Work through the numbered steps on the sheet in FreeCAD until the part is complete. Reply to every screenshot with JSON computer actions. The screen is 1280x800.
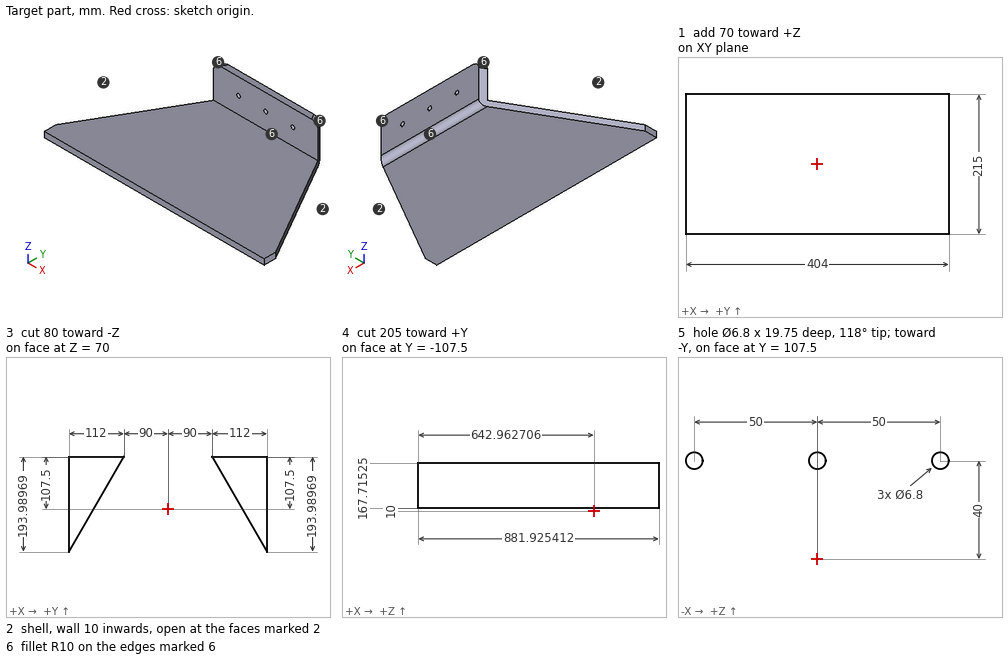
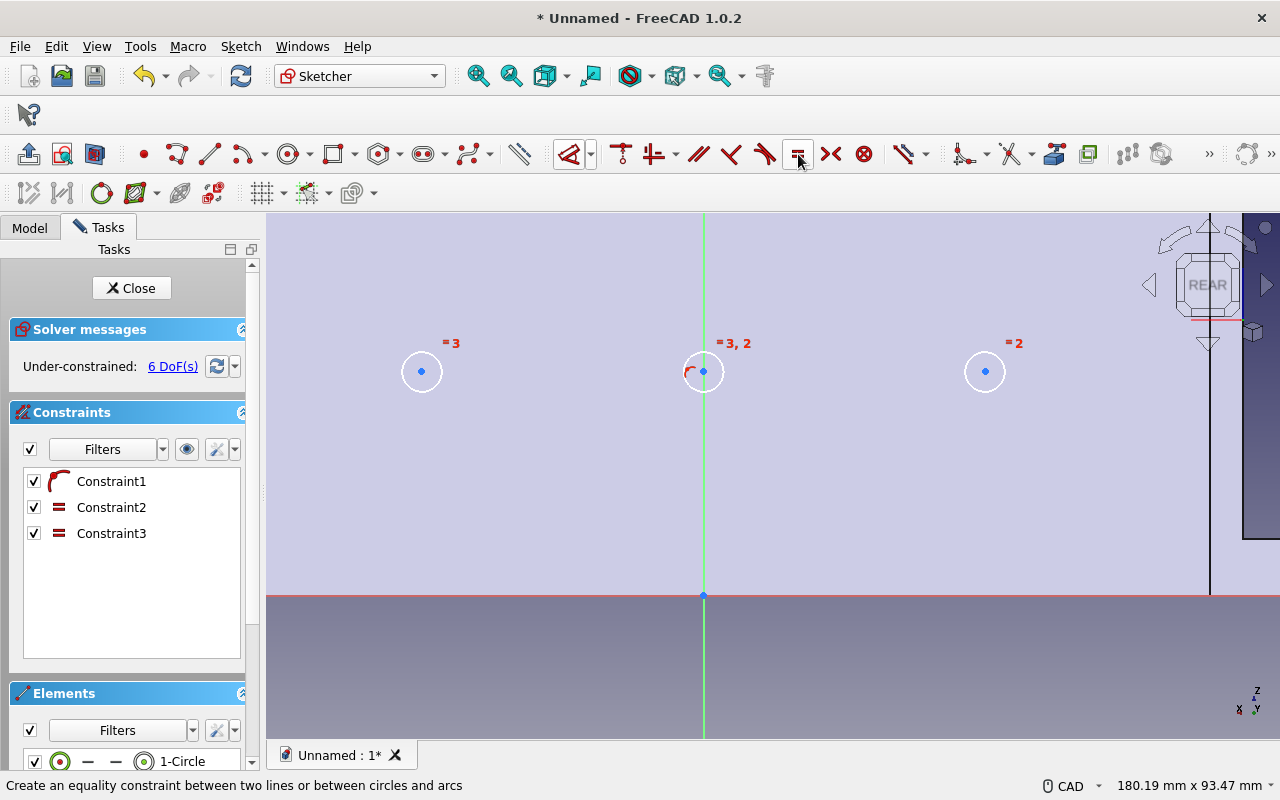
{"action": "left_click", "coordinate": [985, 372]}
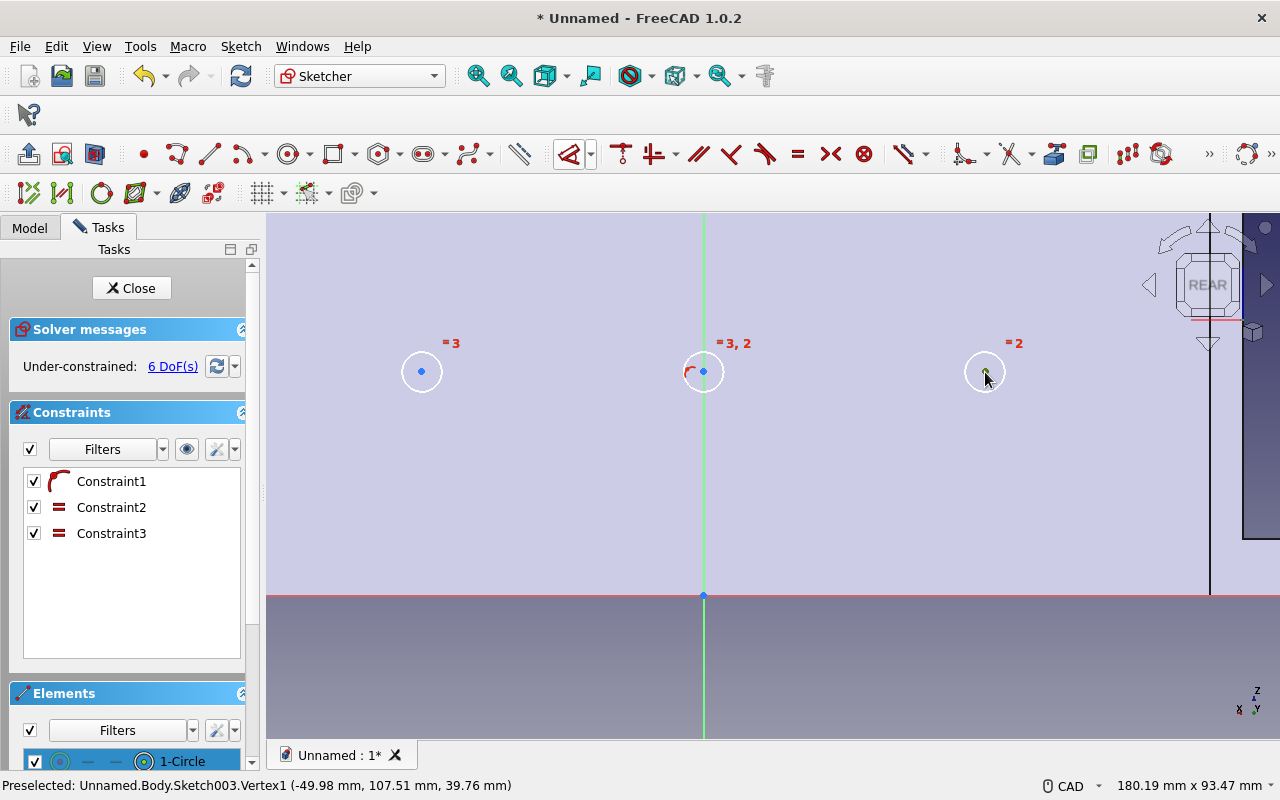
{"action": "left_click", "coordinate": [704, 372]}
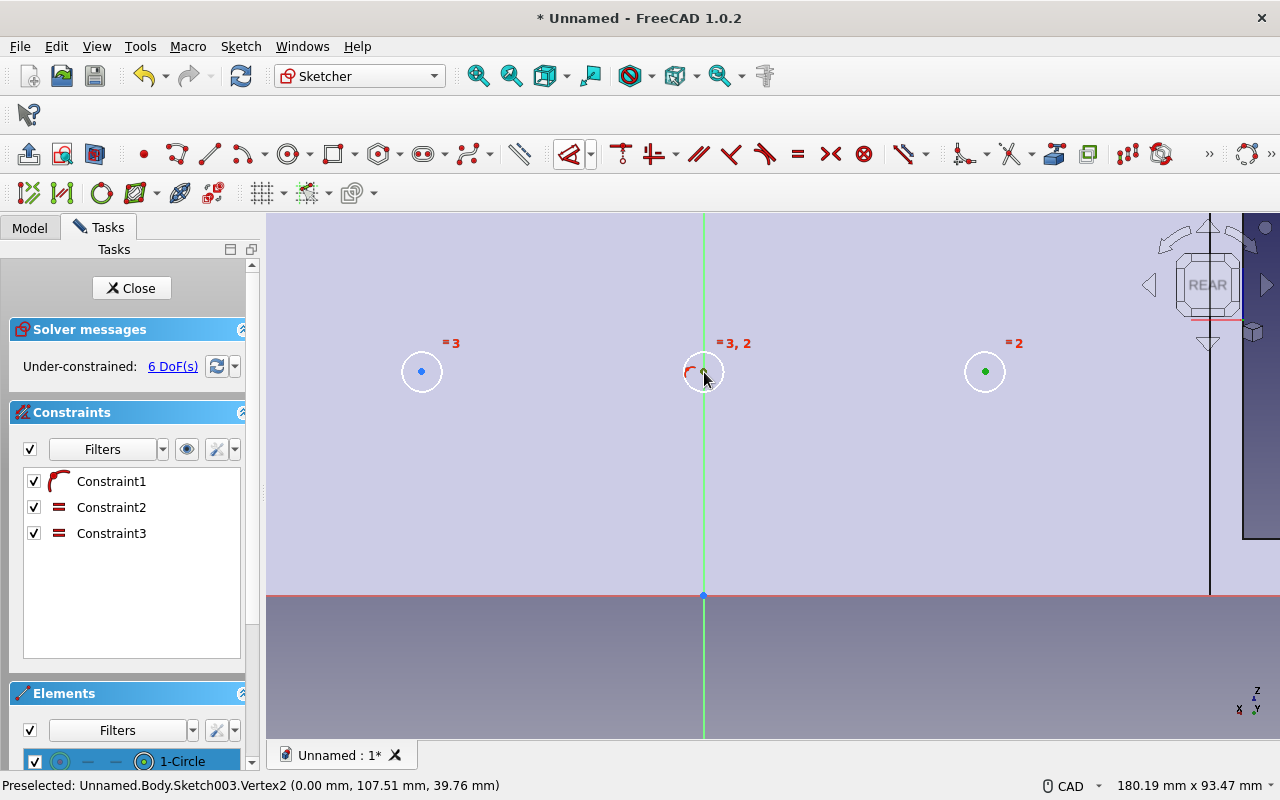
{"action": "left_click", "coordinate": [676, 154]}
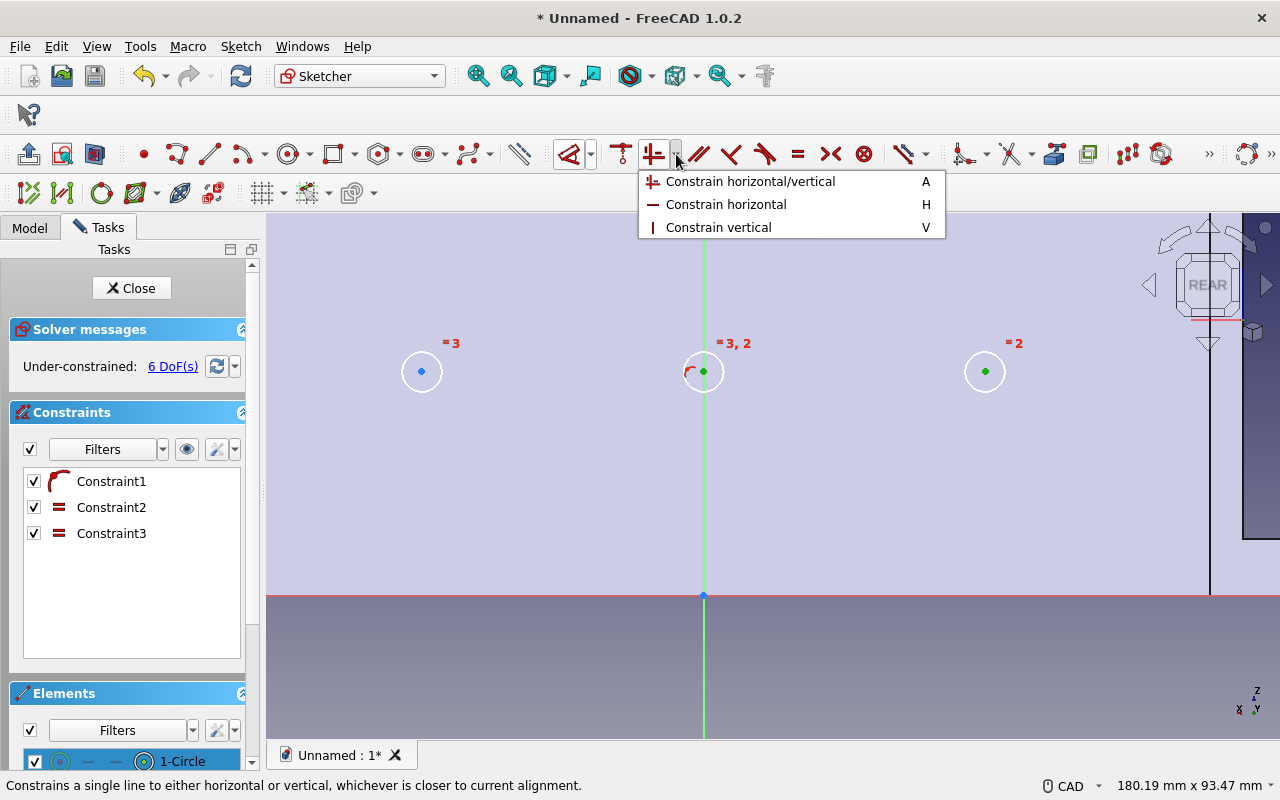
{"action": "left_click", "coordinate": [792, 204]}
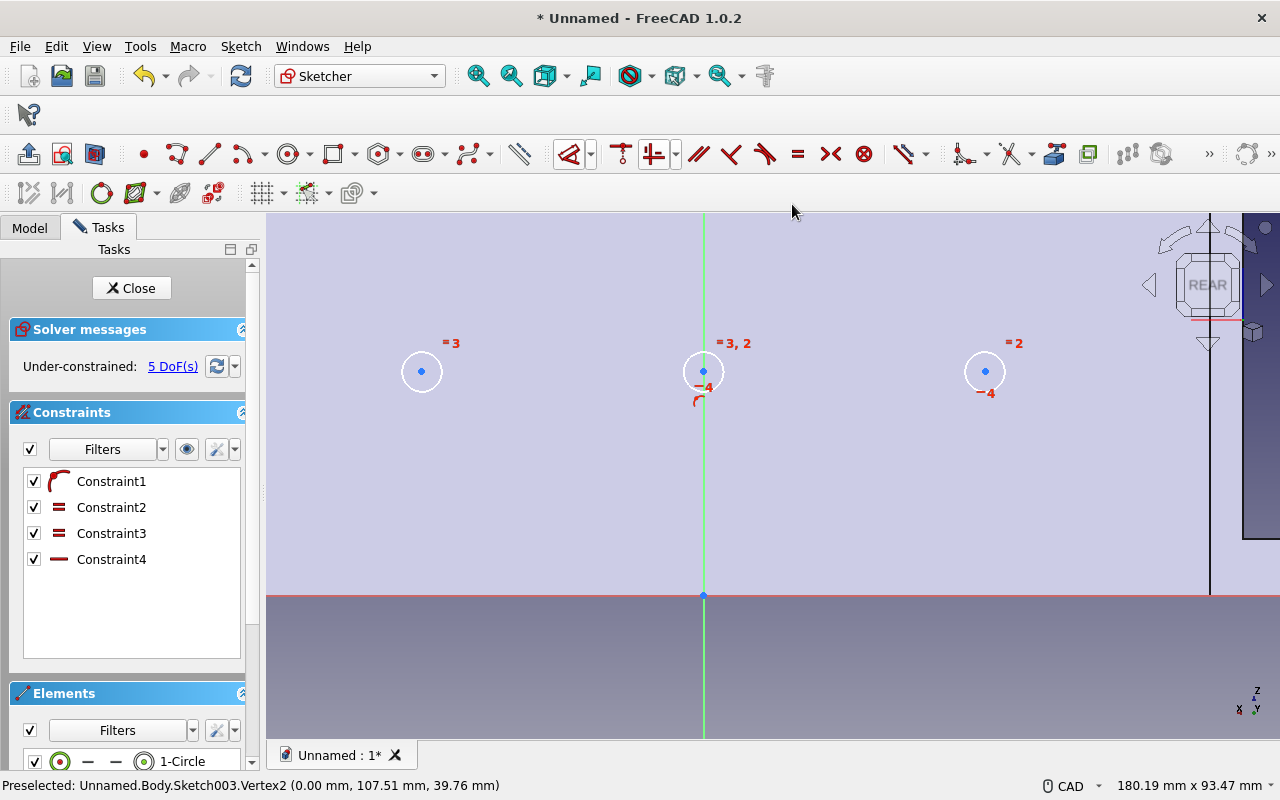
{"action": "left_click", "coordinate": [704, 372]}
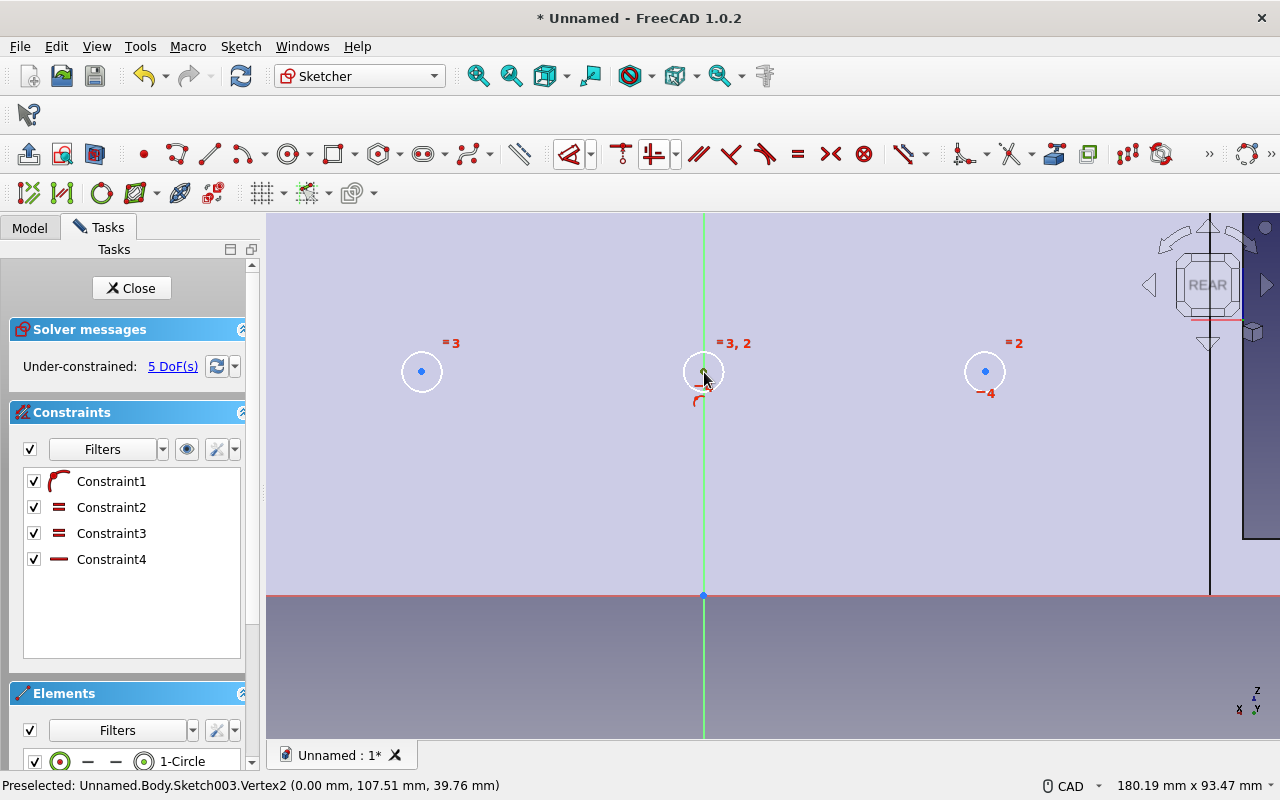
{"action": "left_click", "coordinate": [422, 372]}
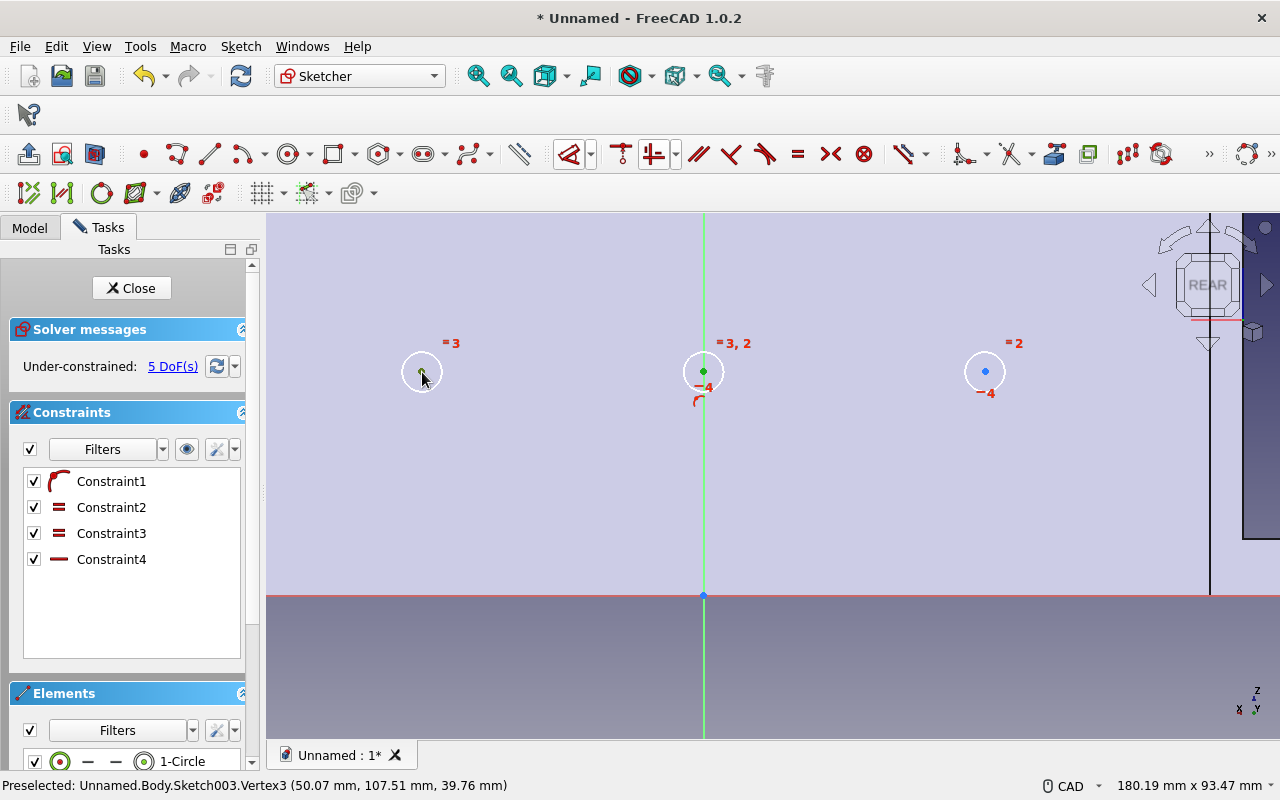
{"action": "left_click", "coordinate": [676, 154]}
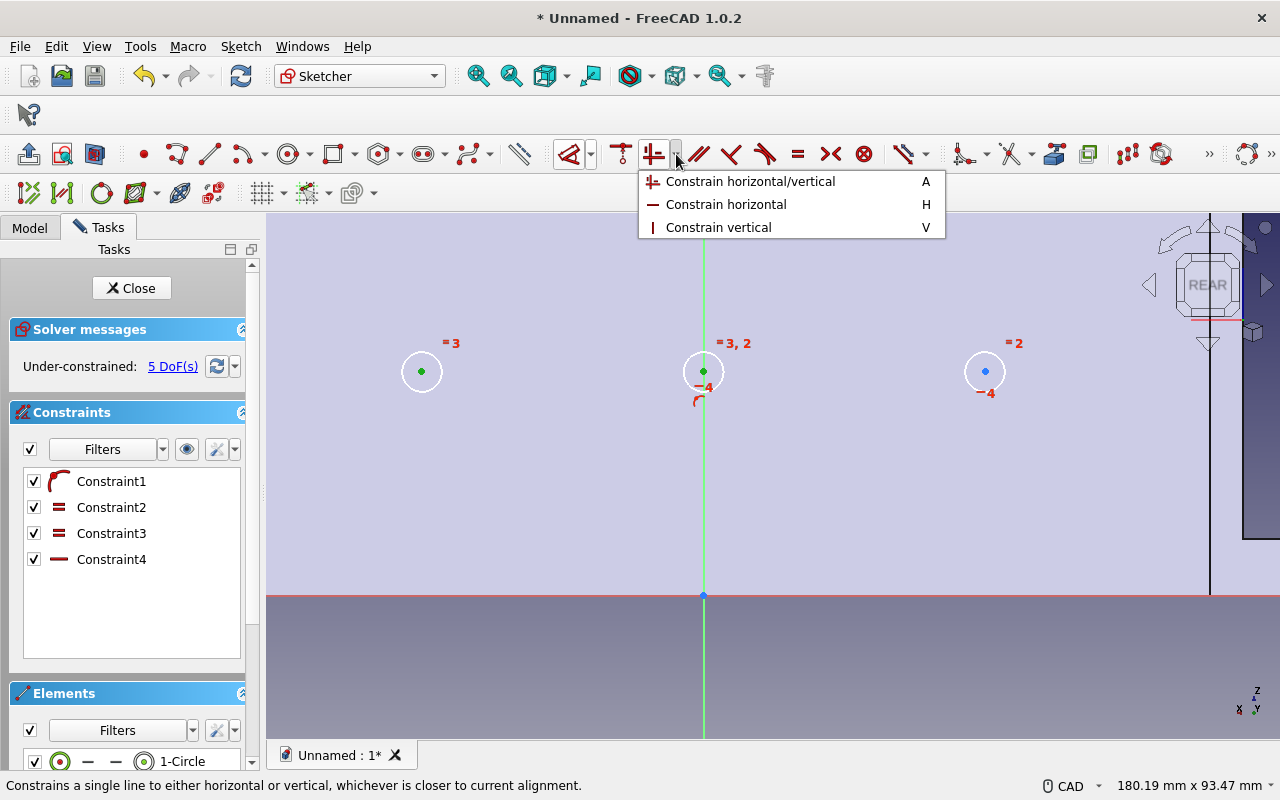
{"action": "left_click", "coordinate": [792, 204]}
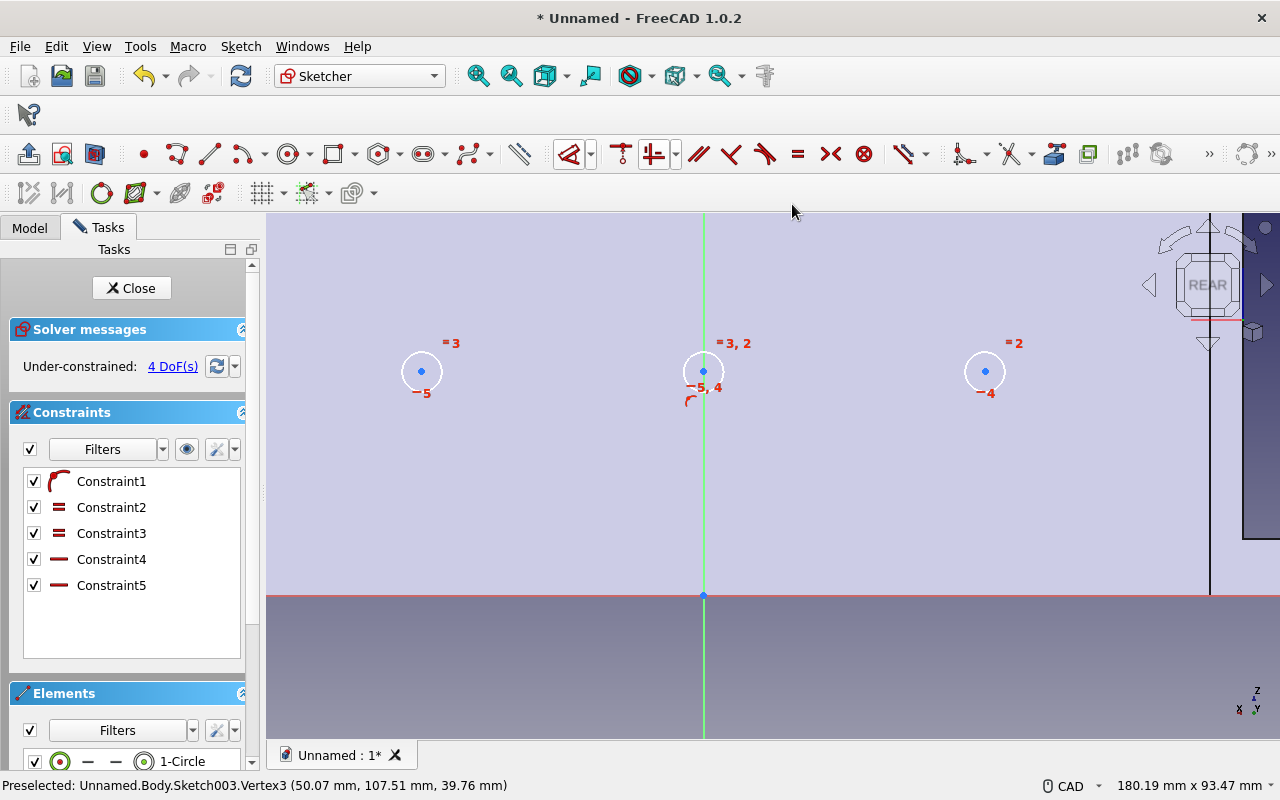
{"action": "left_click", "coordinate": [999, 358]}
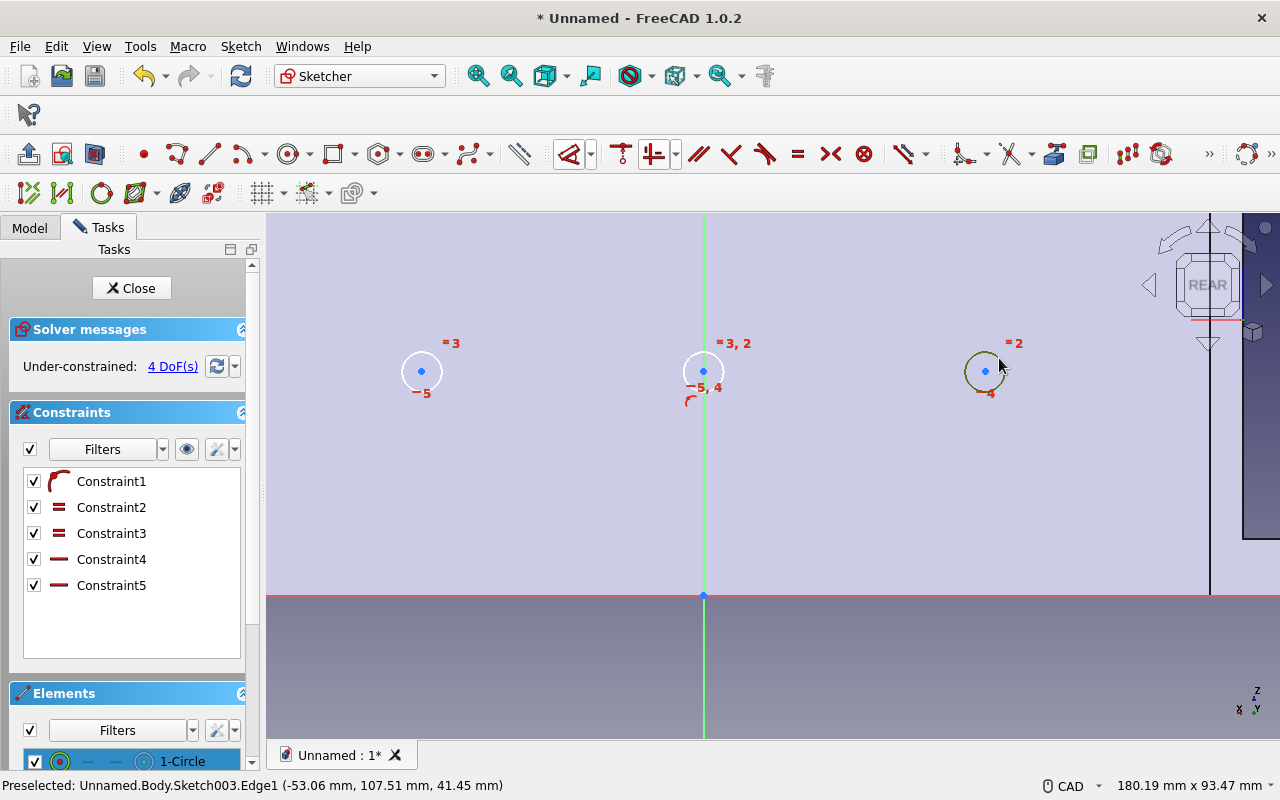
{"action": "left_click", "coordinate": [590, 154]}